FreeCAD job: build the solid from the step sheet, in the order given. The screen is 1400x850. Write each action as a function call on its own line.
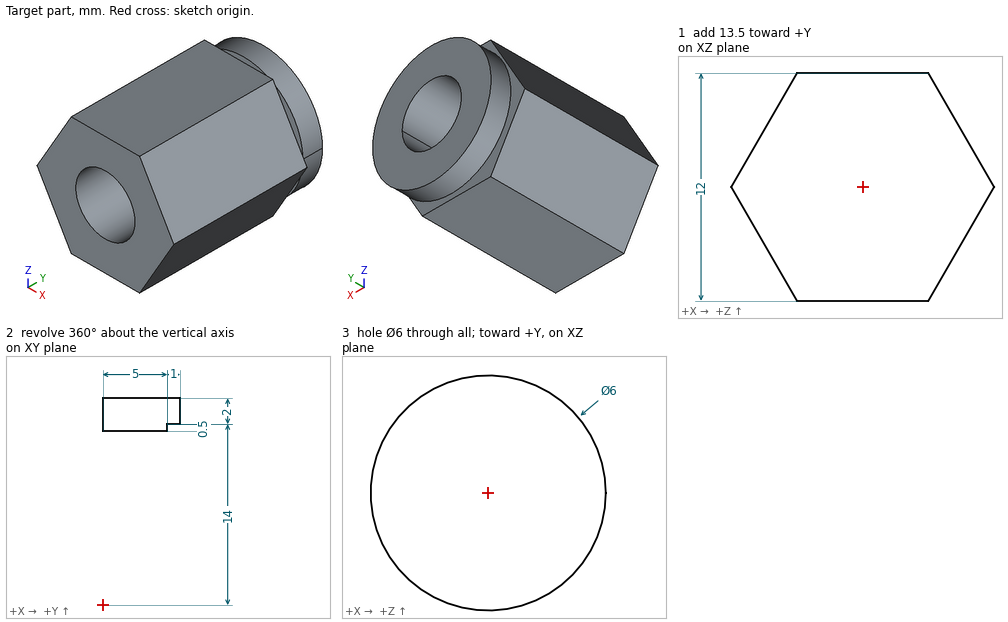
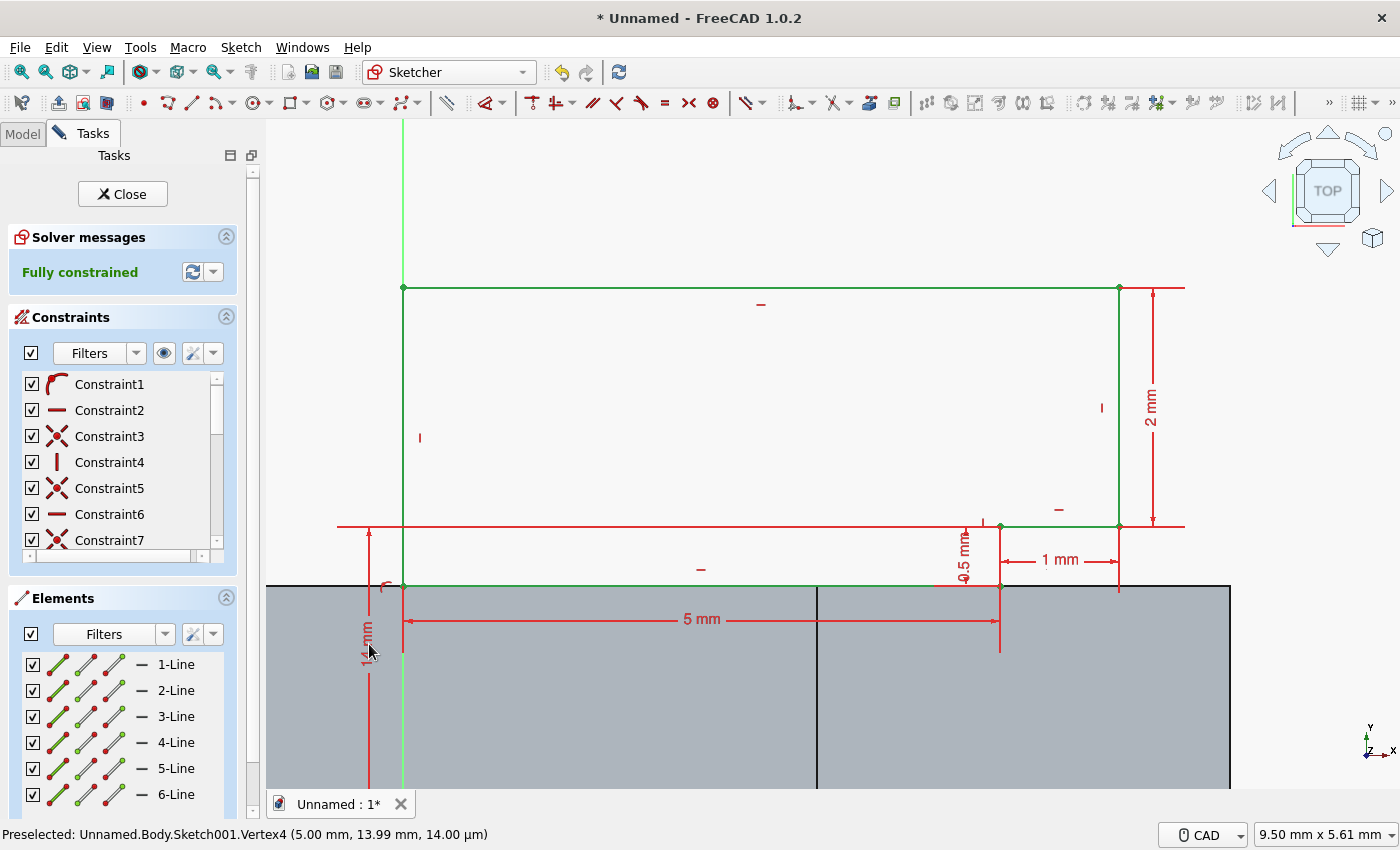
click(123, 194)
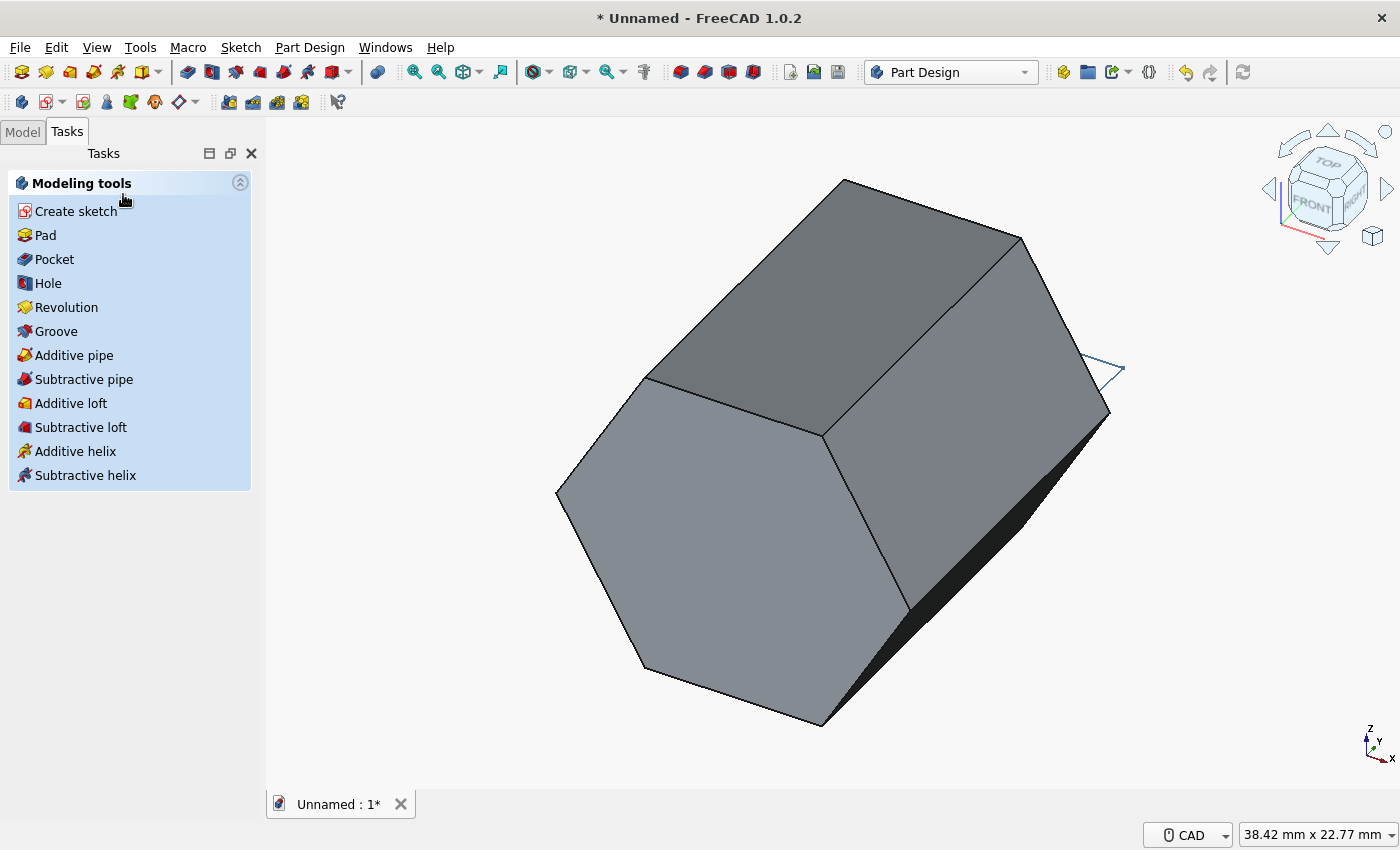
click(46, 72)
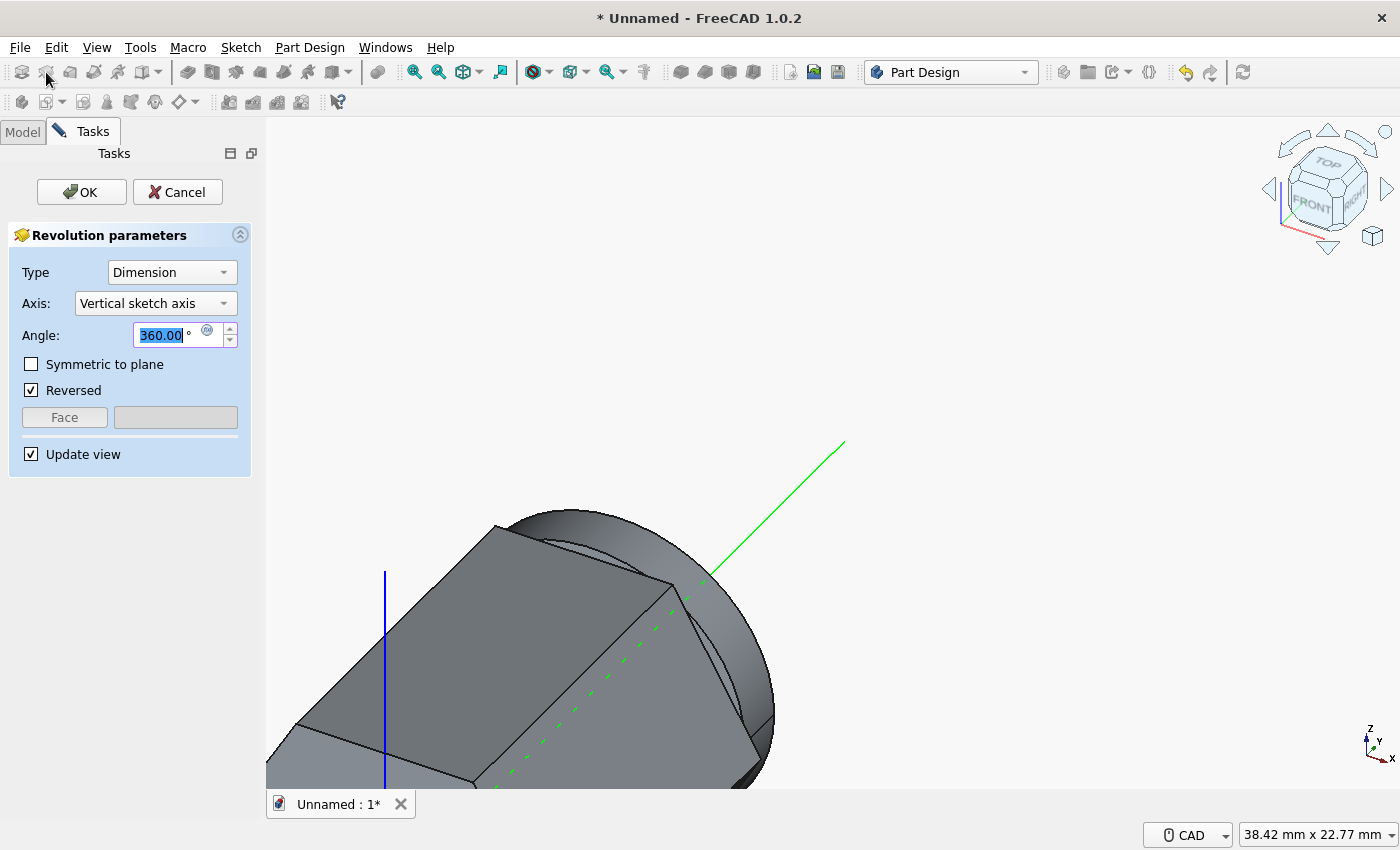
click(82, 192)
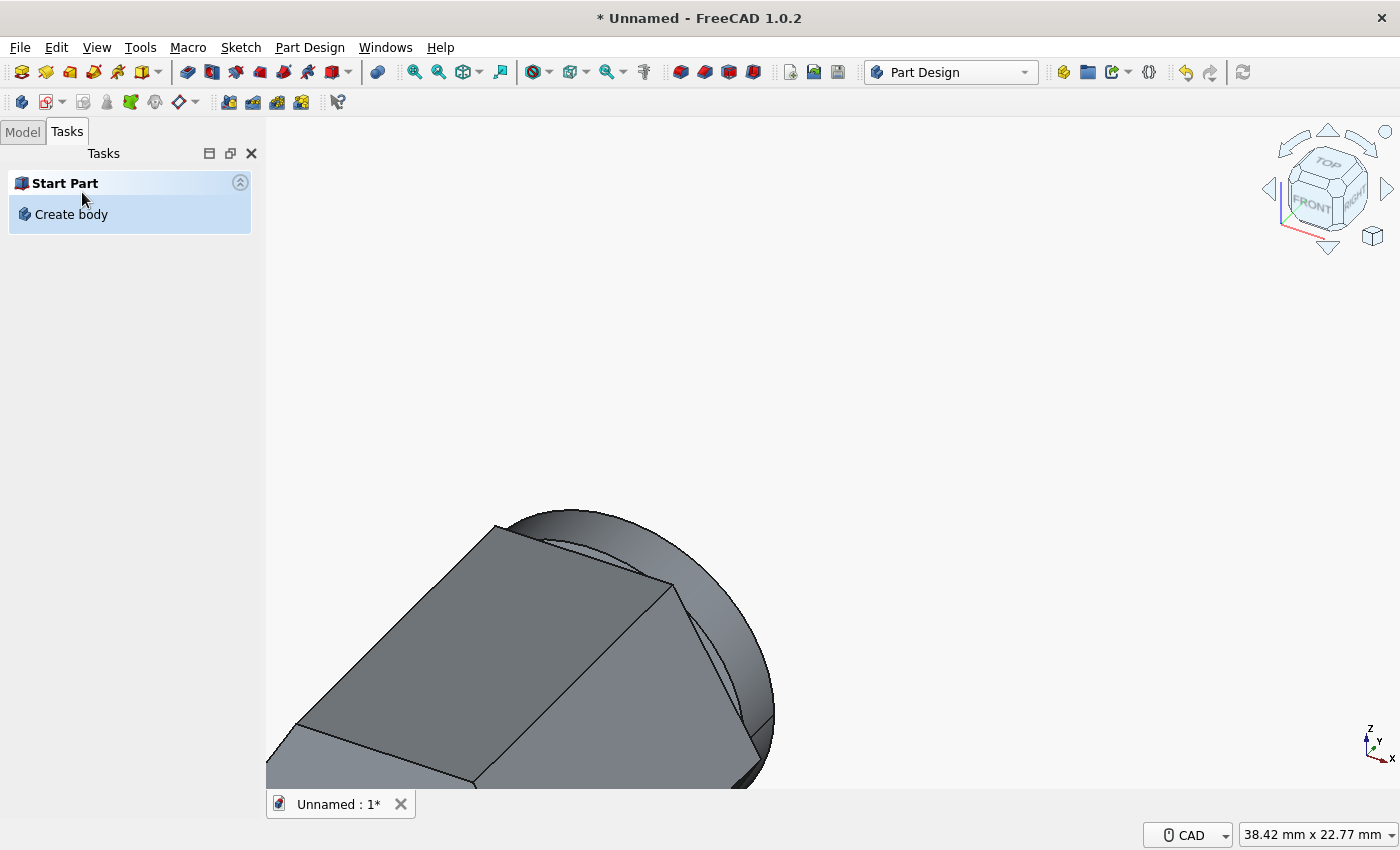
click(416, 72)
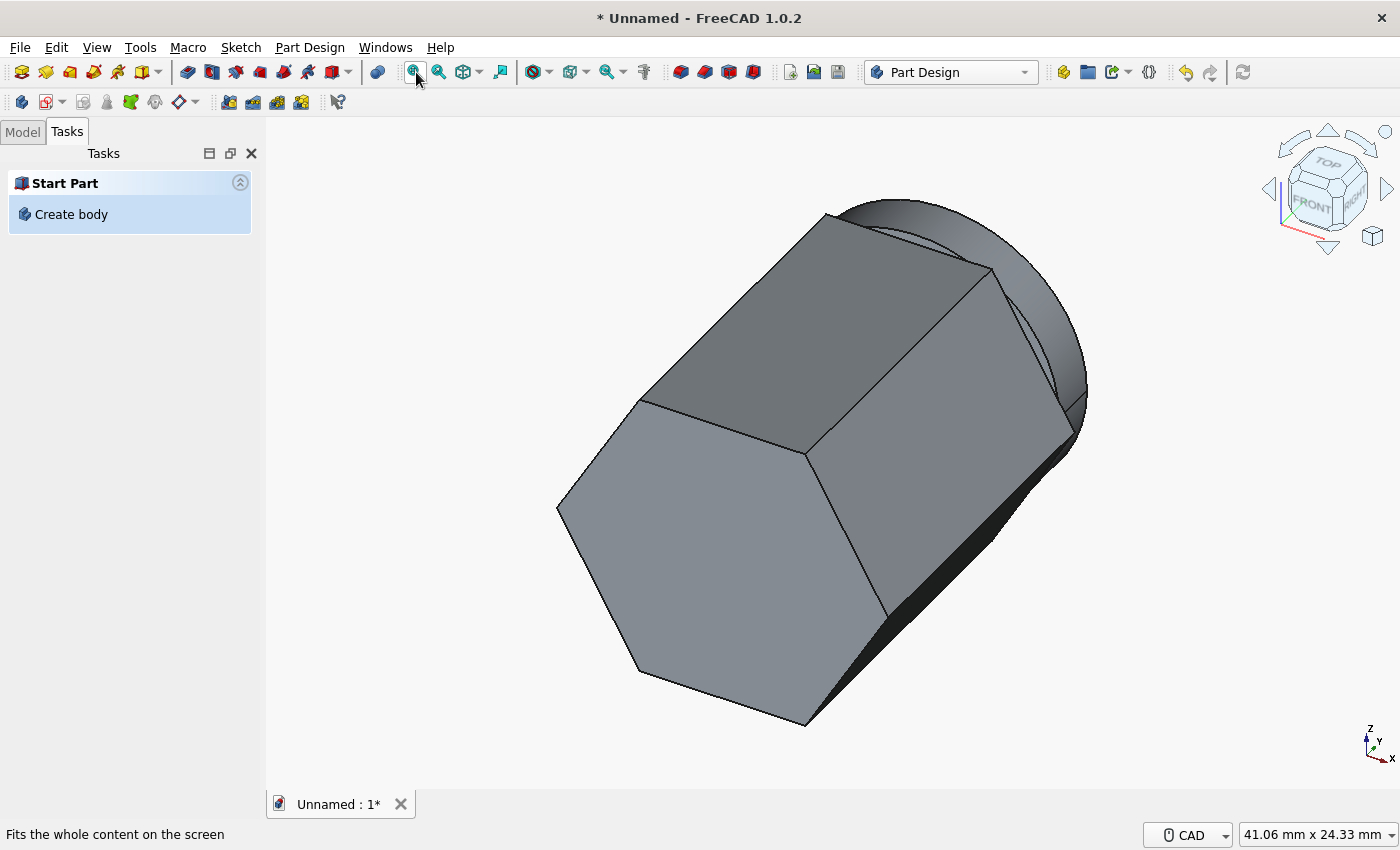
click(46, 102)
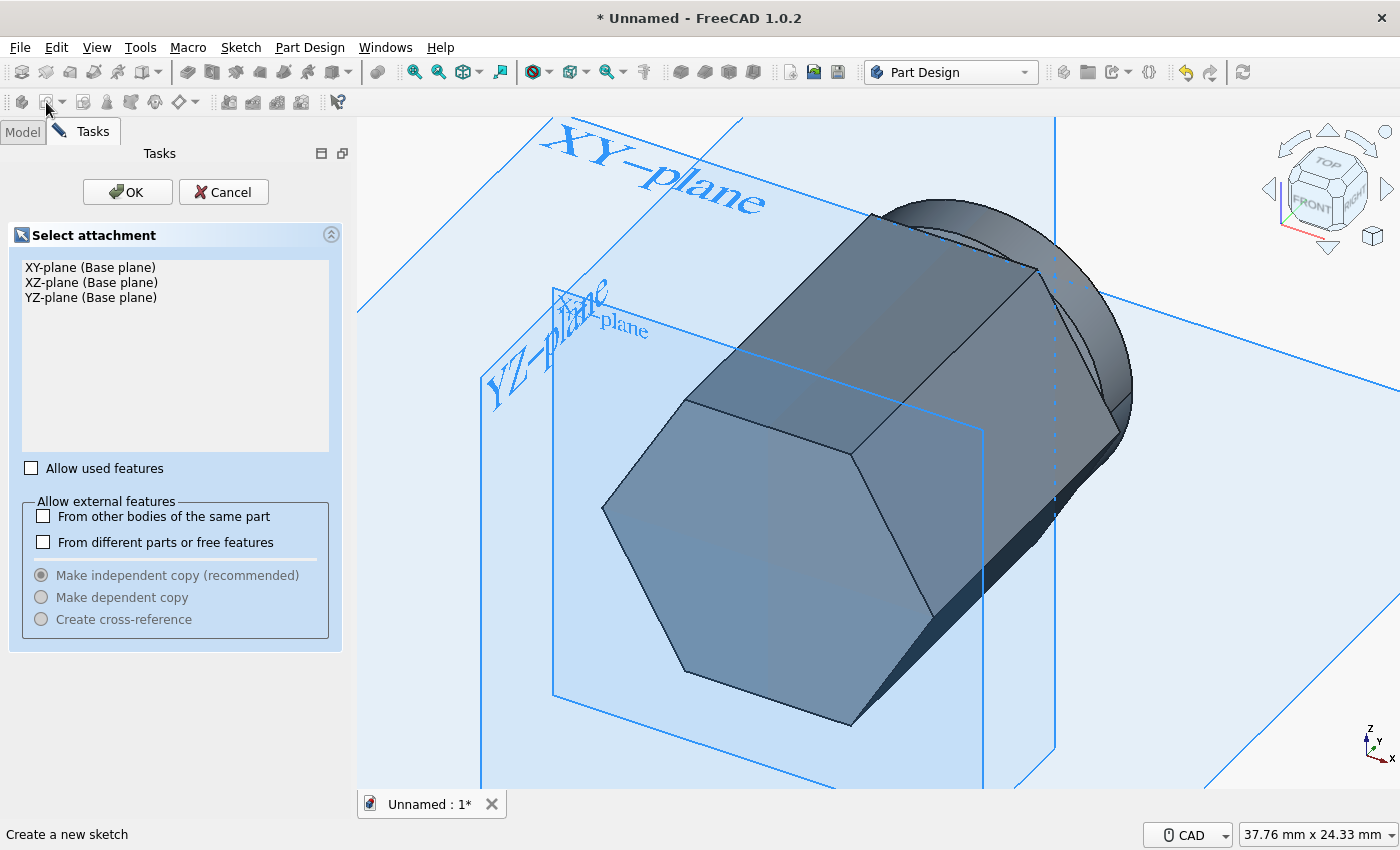
click(82, 282)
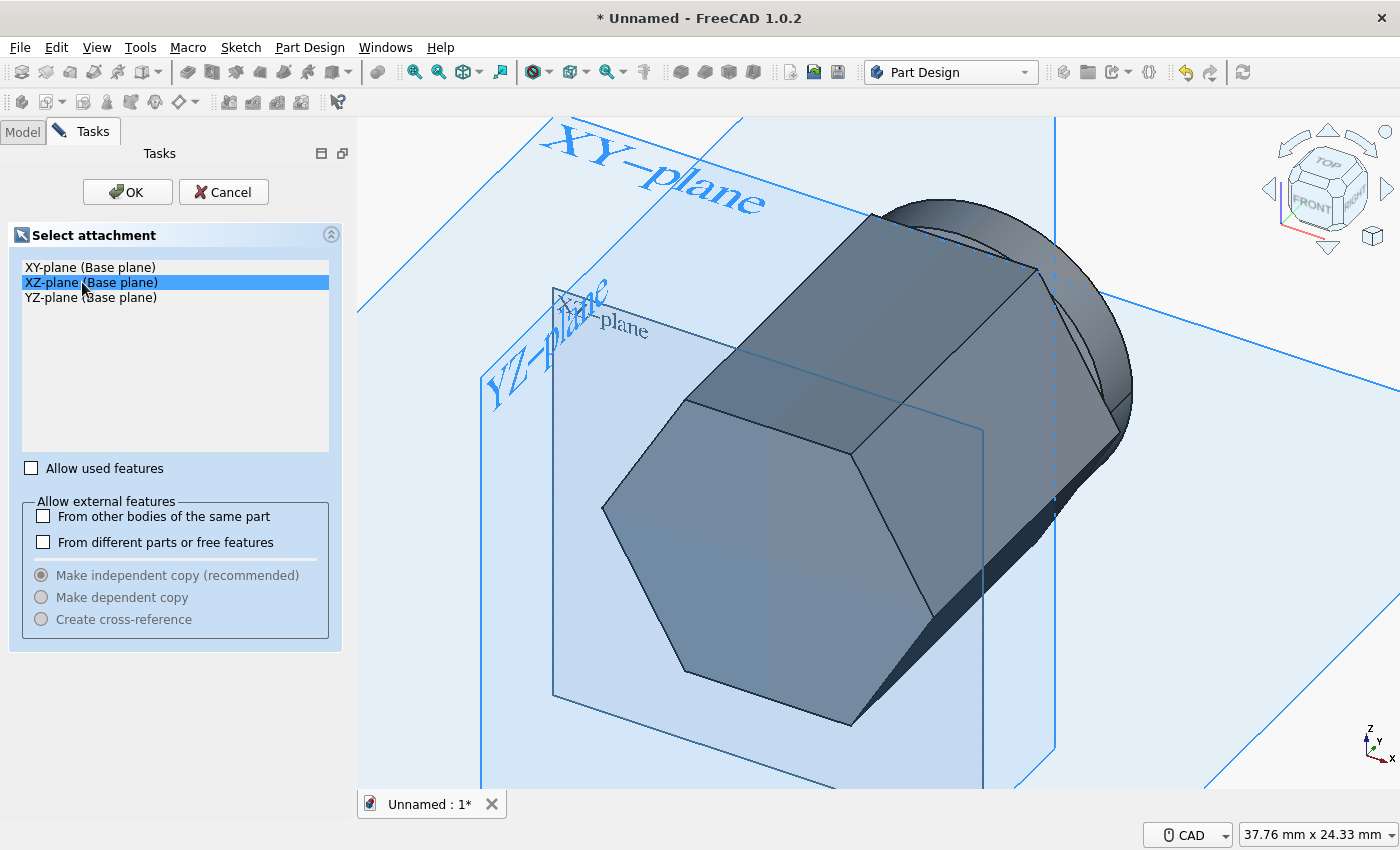
click(128, 192)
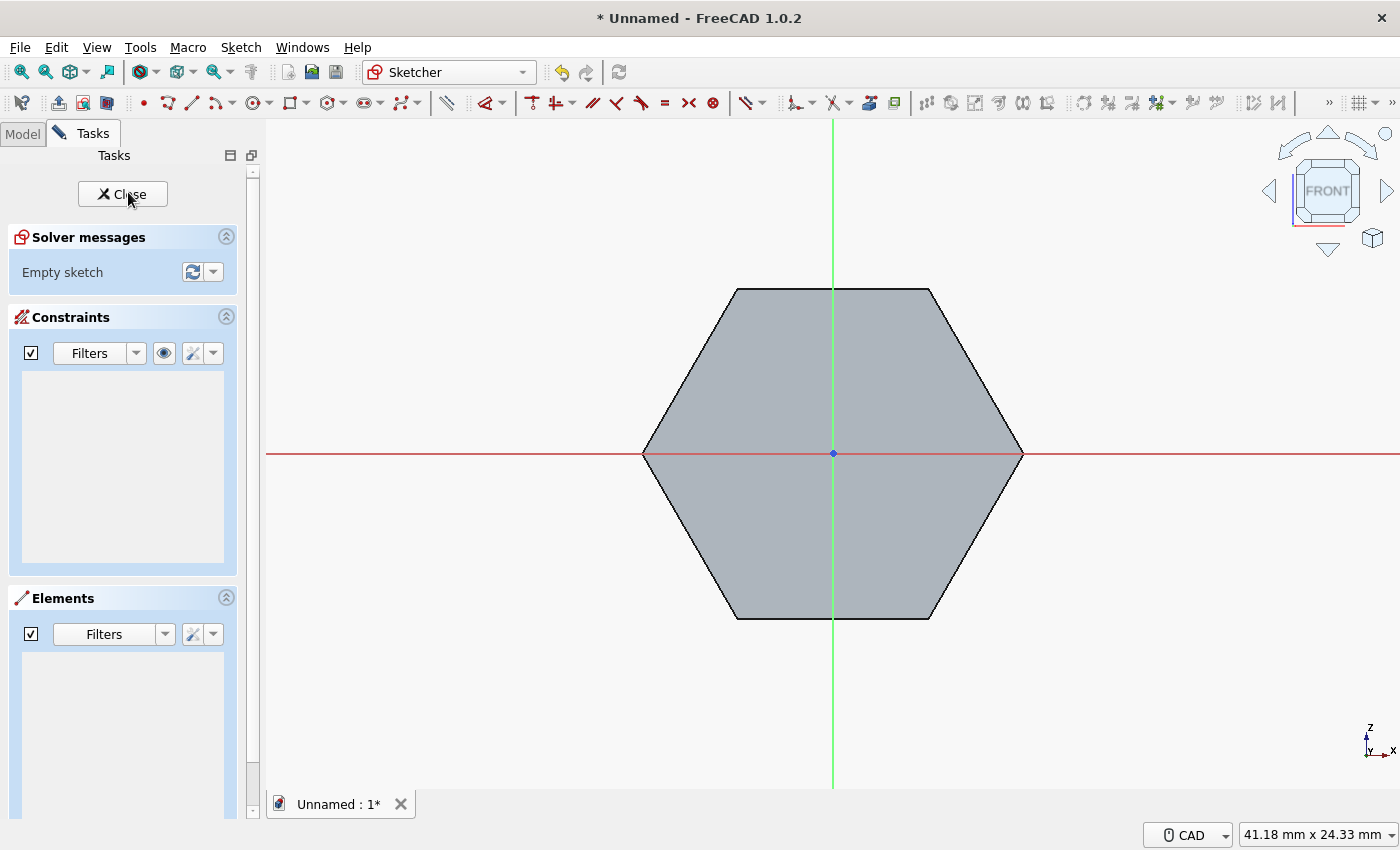
scroll(873, 454, up, 5)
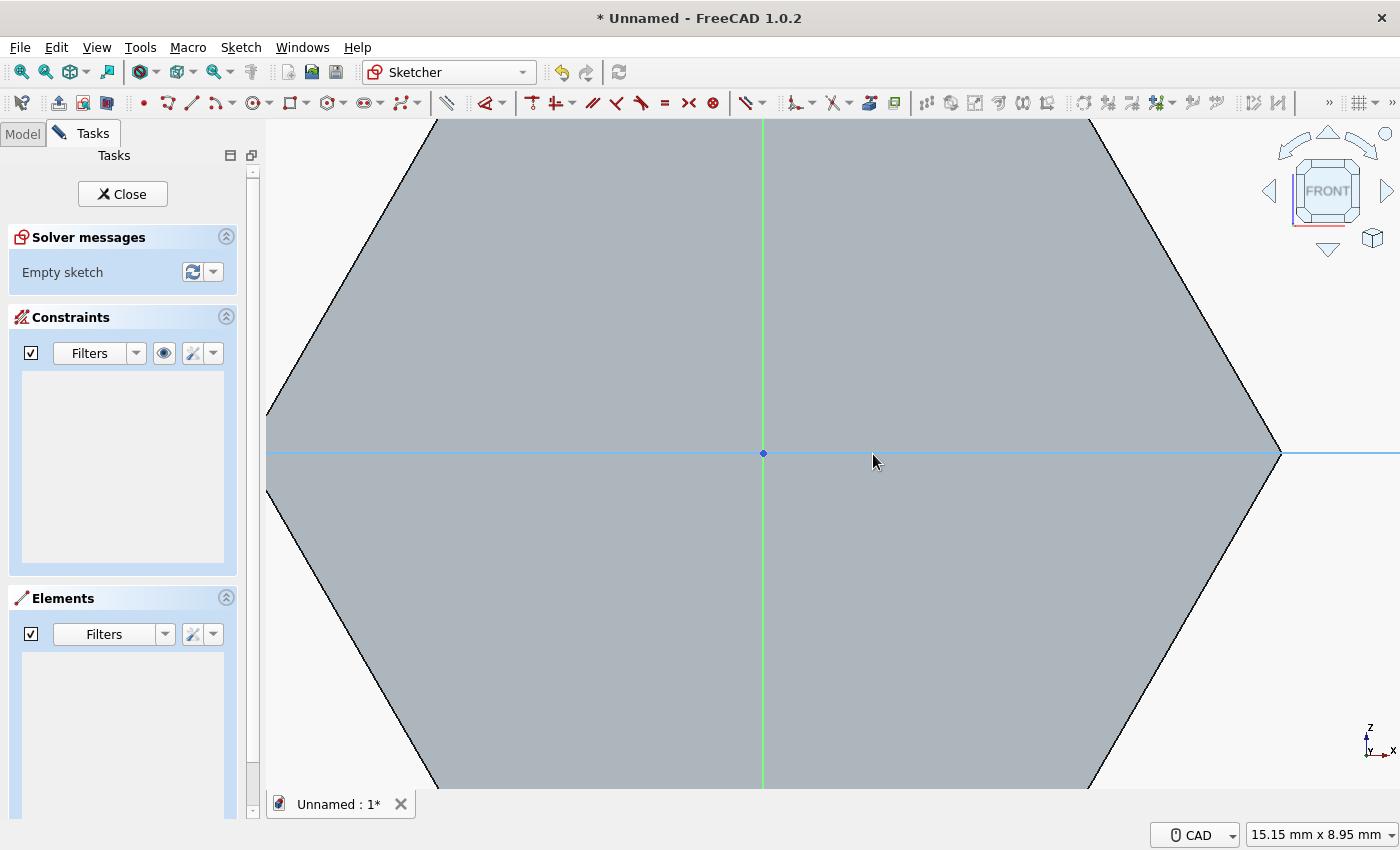
click(254, 104)